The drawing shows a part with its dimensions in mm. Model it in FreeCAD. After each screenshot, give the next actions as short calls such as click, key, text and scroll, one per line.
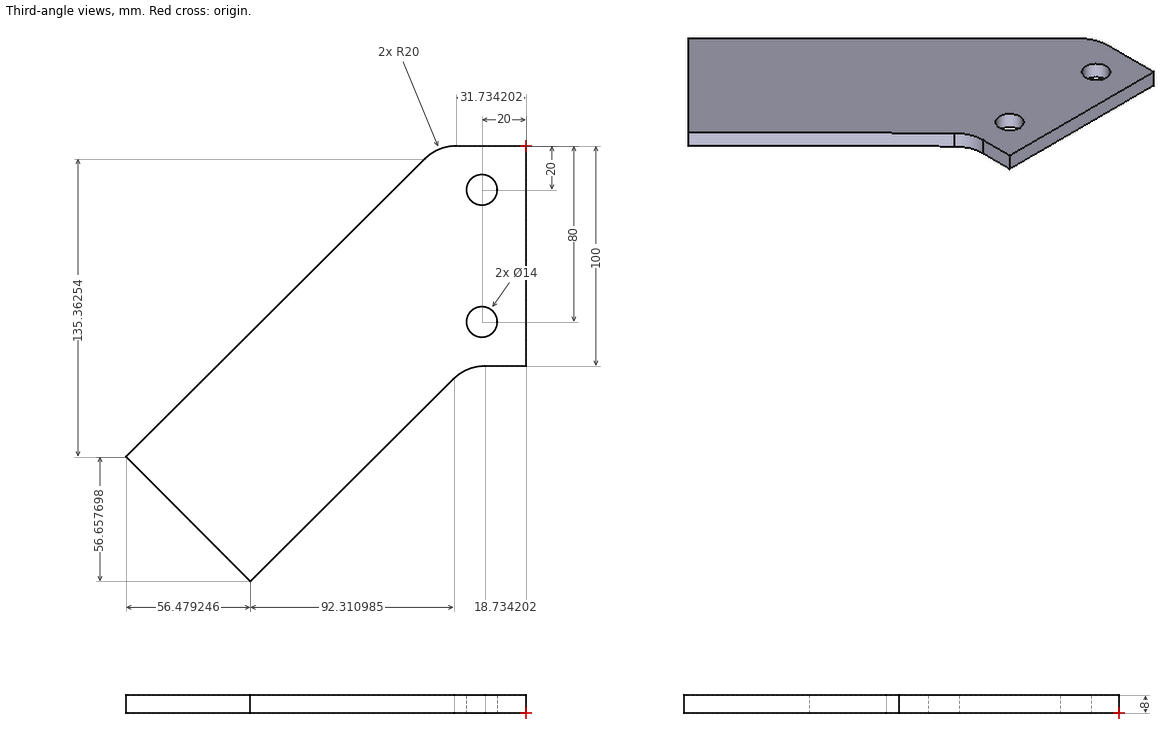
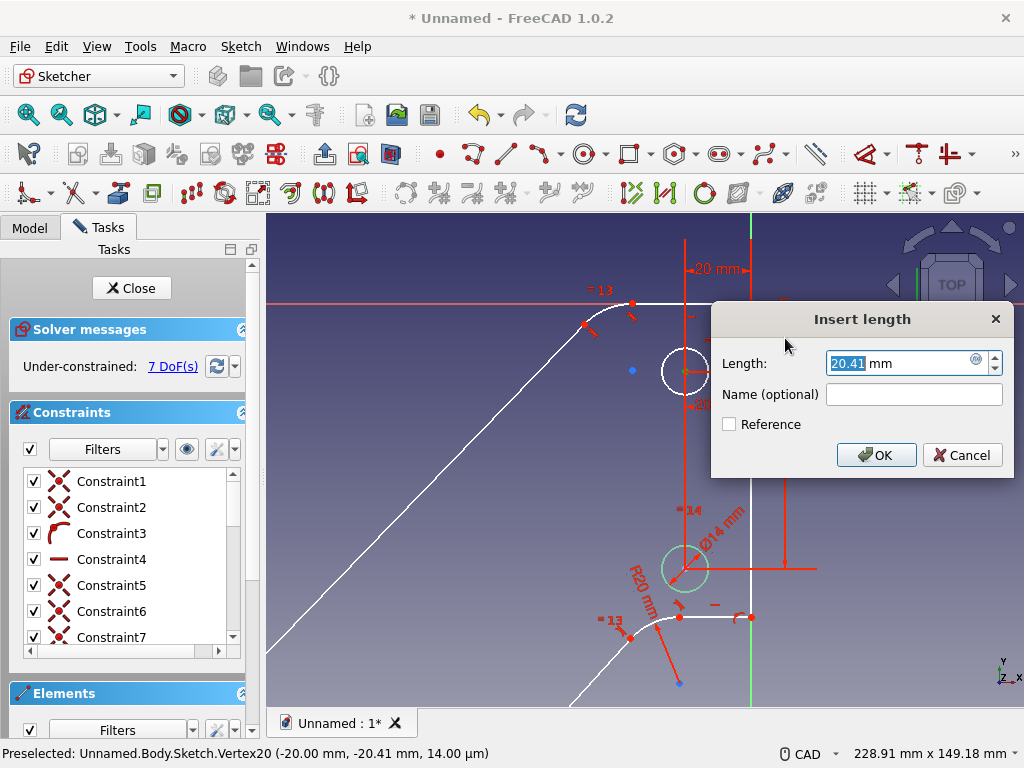
text(20)
key(Return)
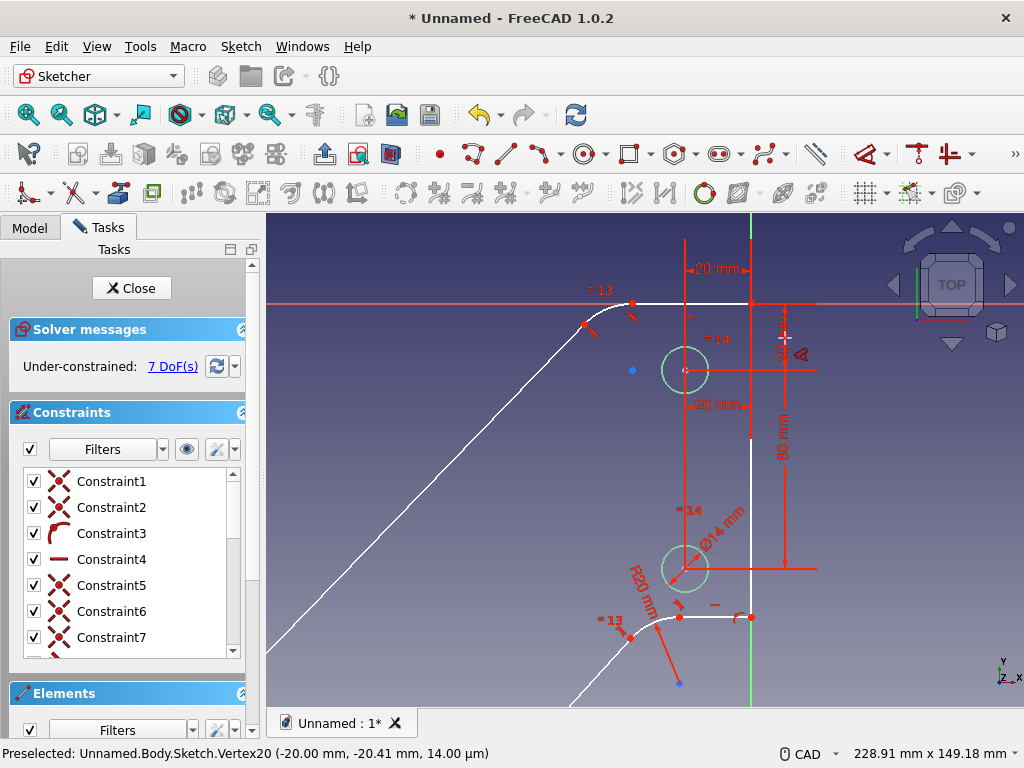
click(751, 523)
click(785, 461)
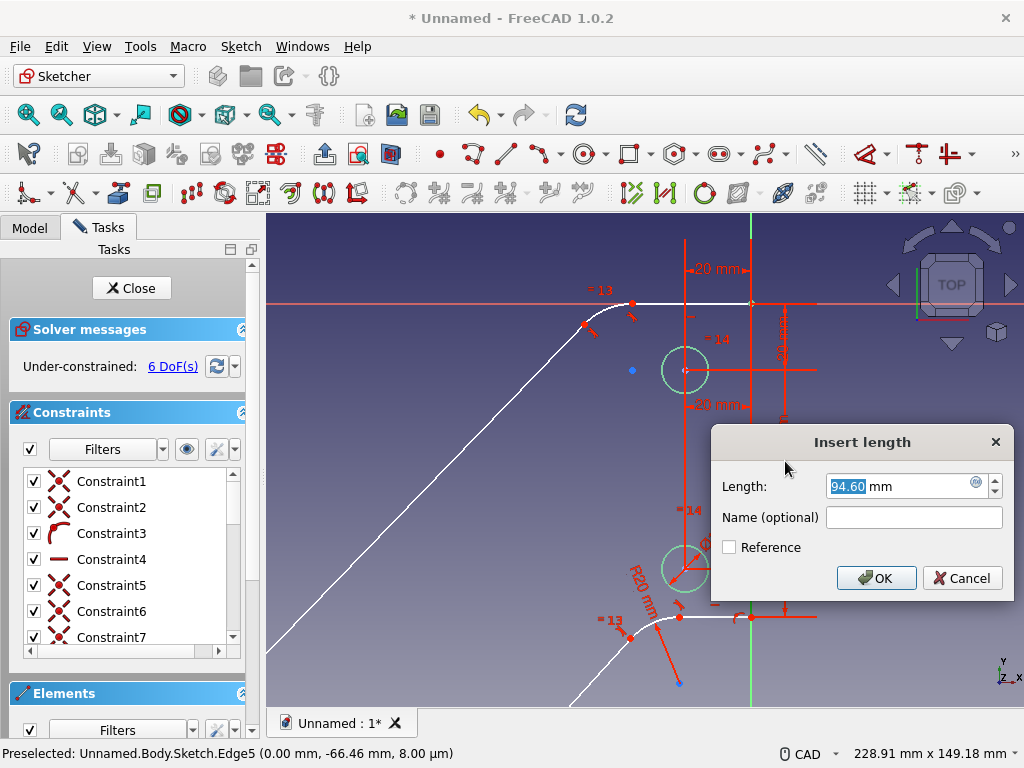
text(100)
key(Return)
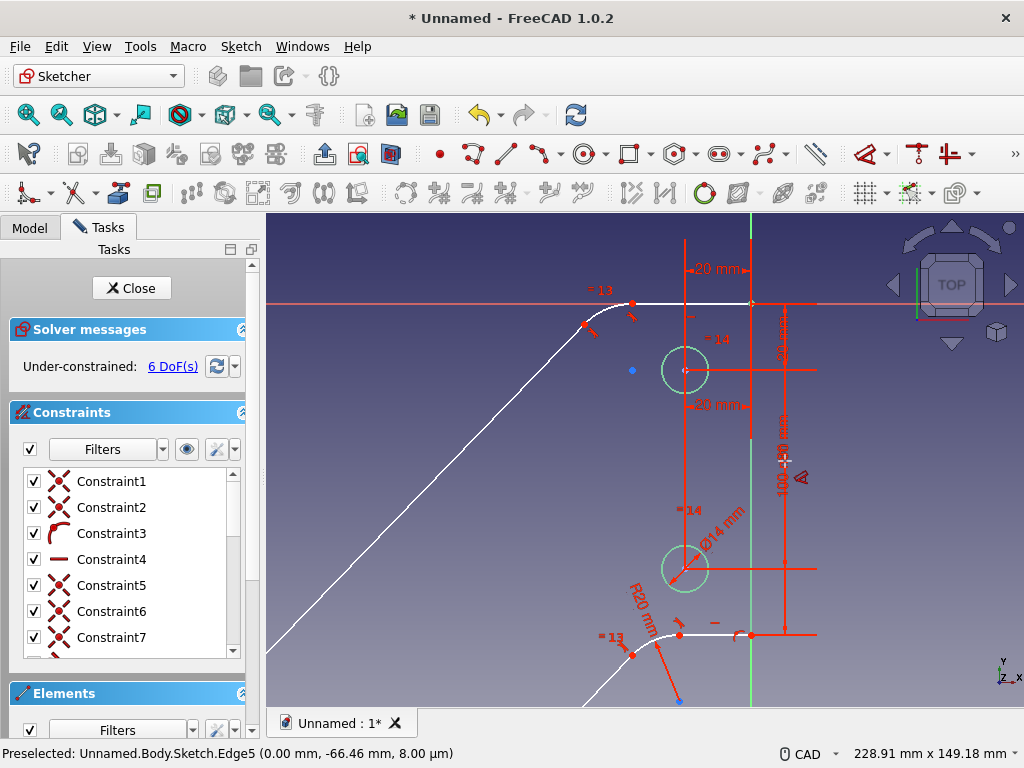
click(701, 635)
click(716, 669)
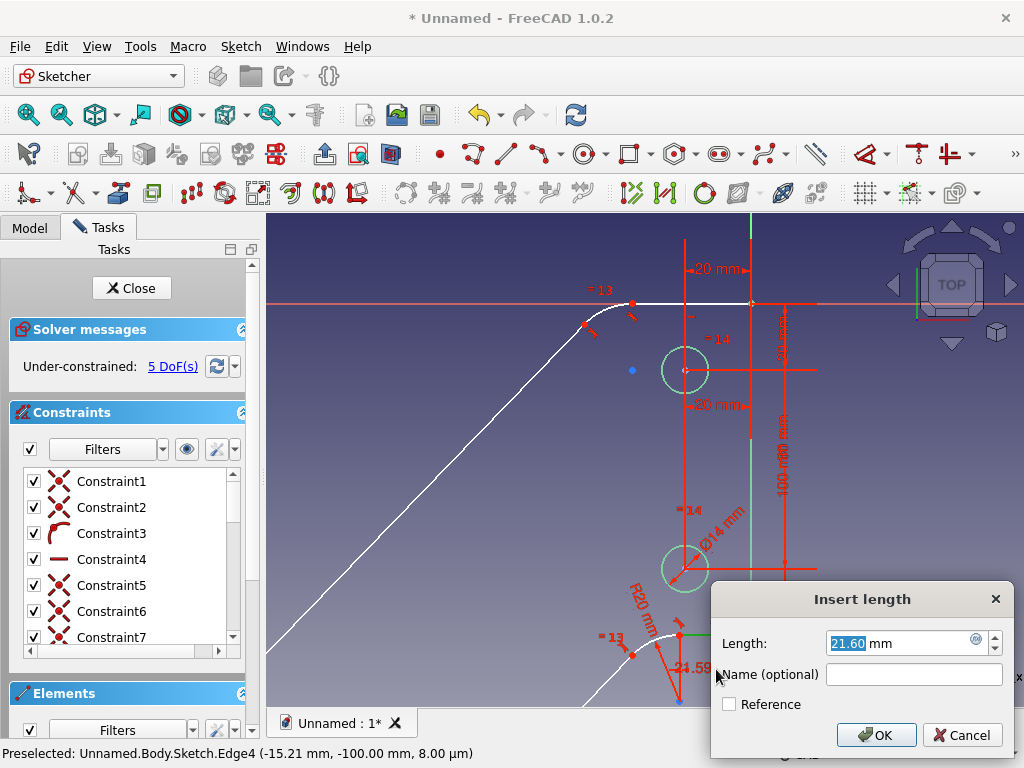
text(18.734202)
key(Return)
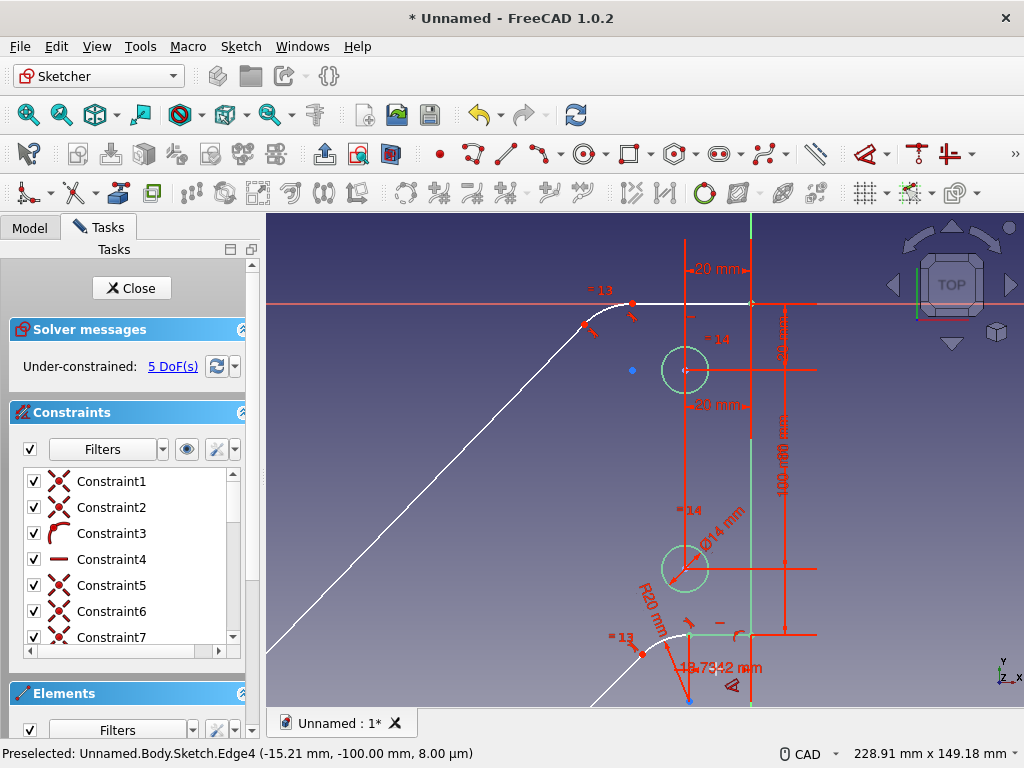
click(716, 304)
click(664, 338)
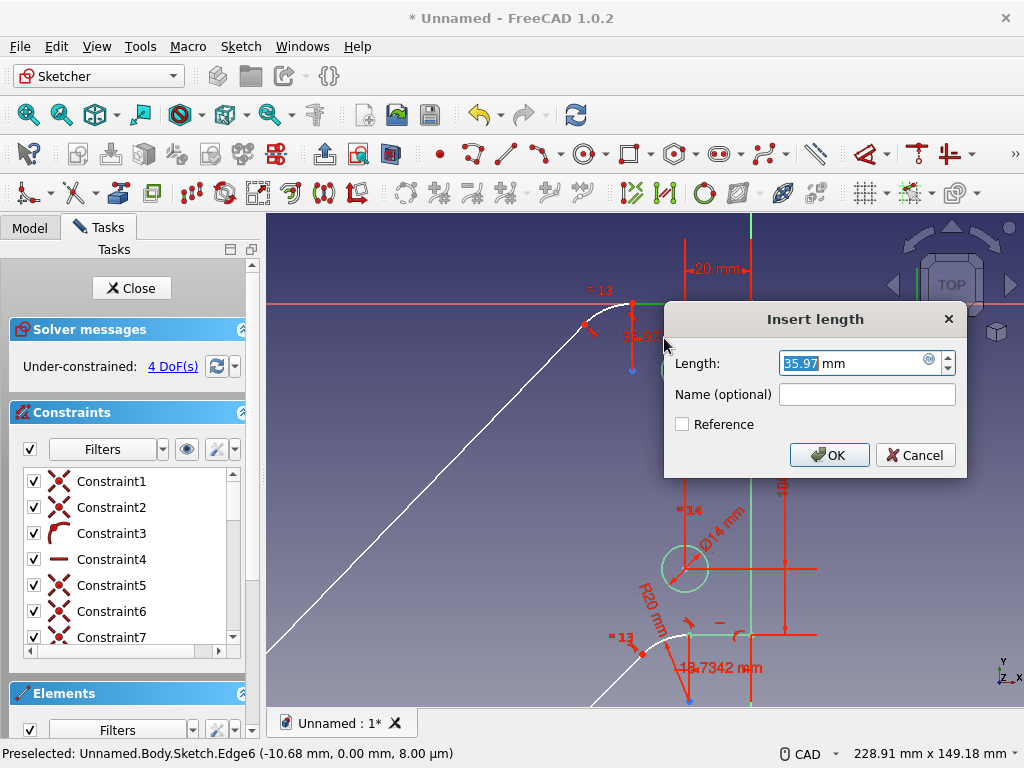
text(31.734202)
key(Return)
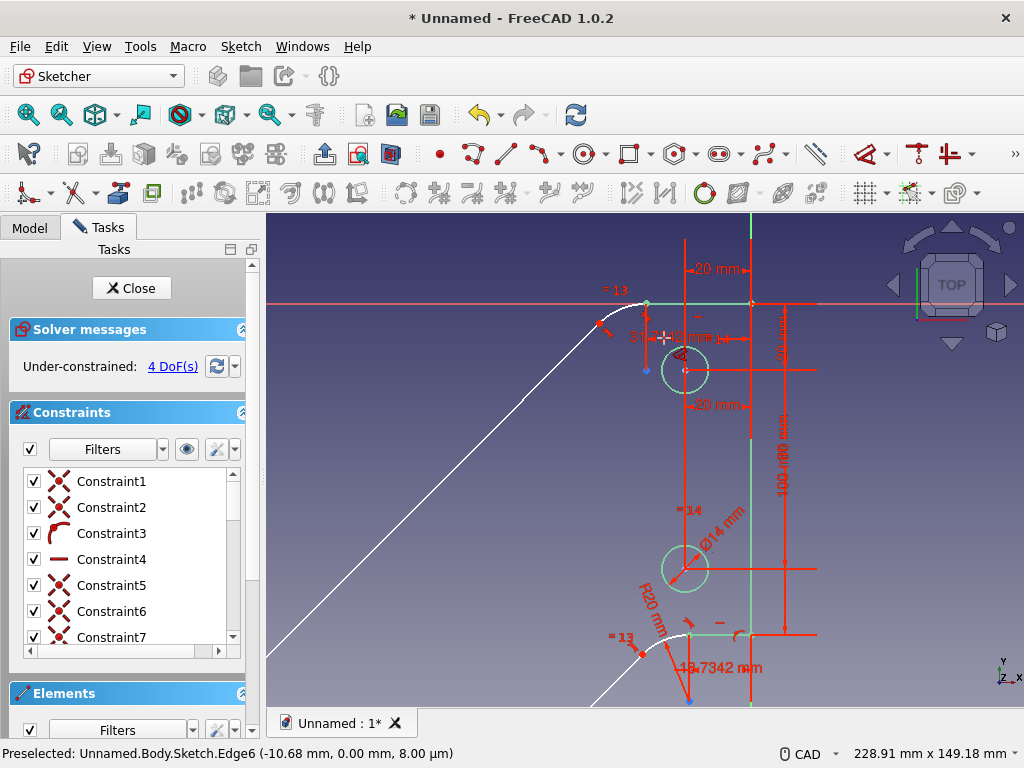
click(465, 458)
click(633, 501)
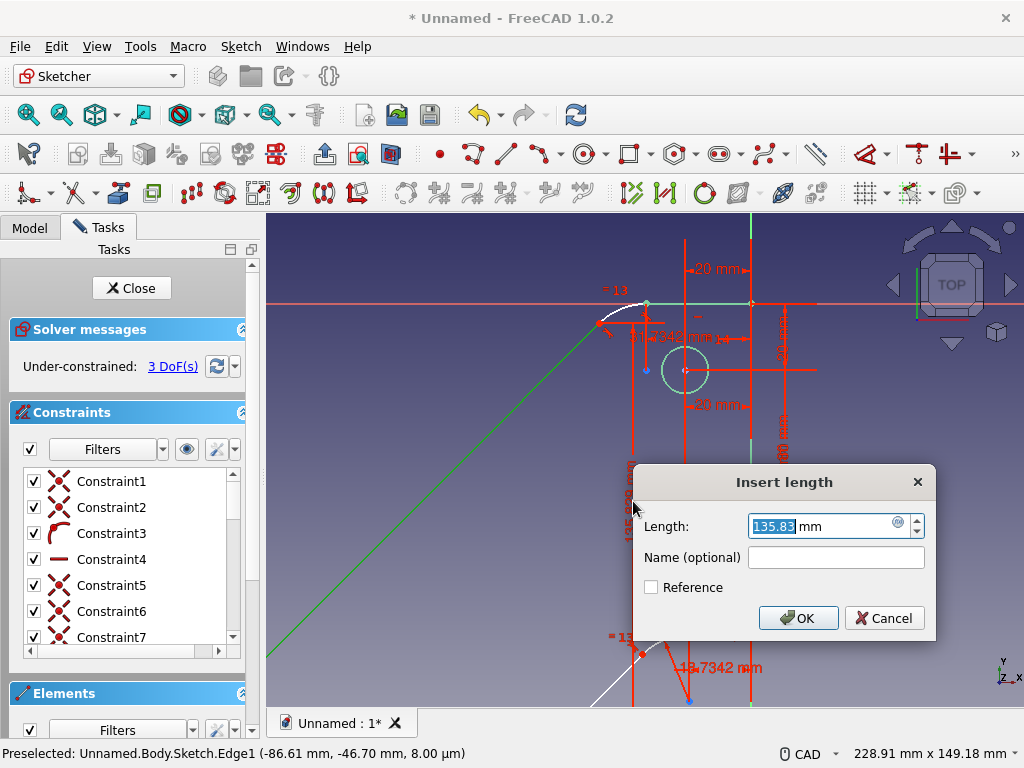
text(135.36254)
key(Return)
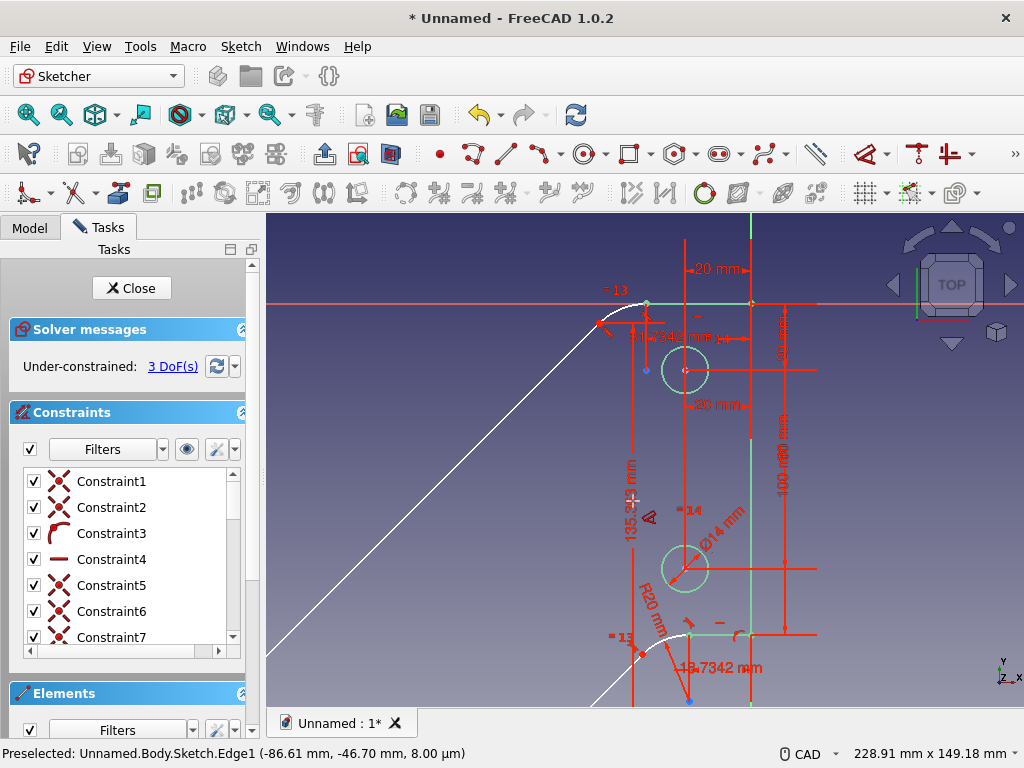
scroll(679, 320, down, 4)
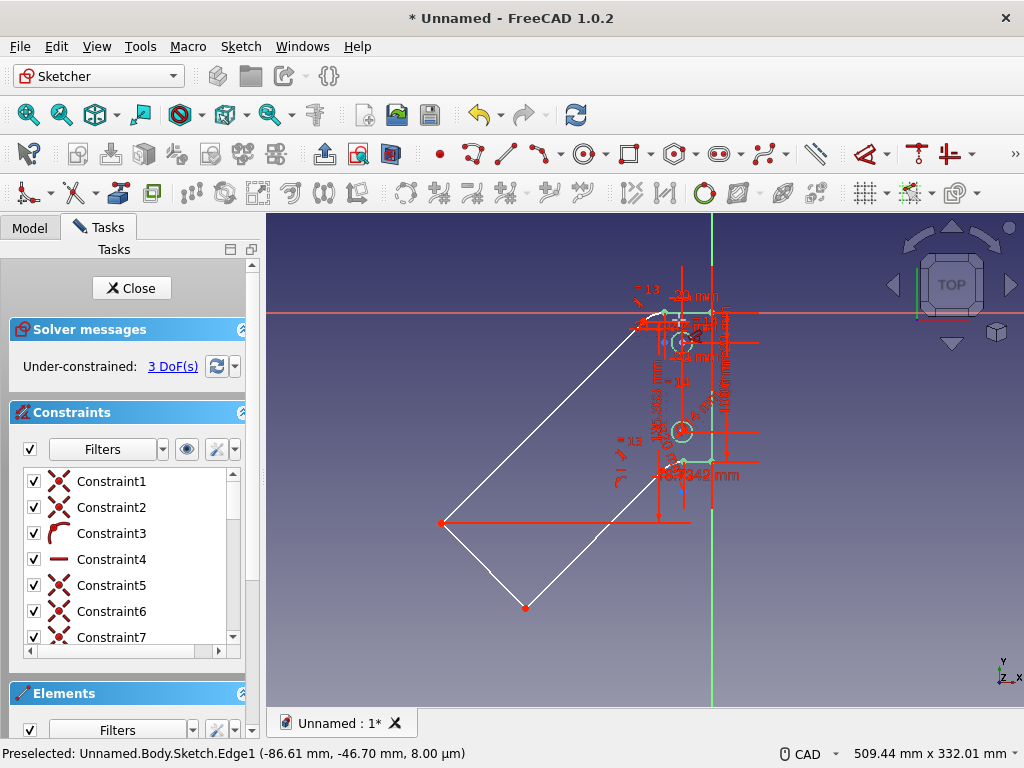
click(467, 549)
click(484, 643)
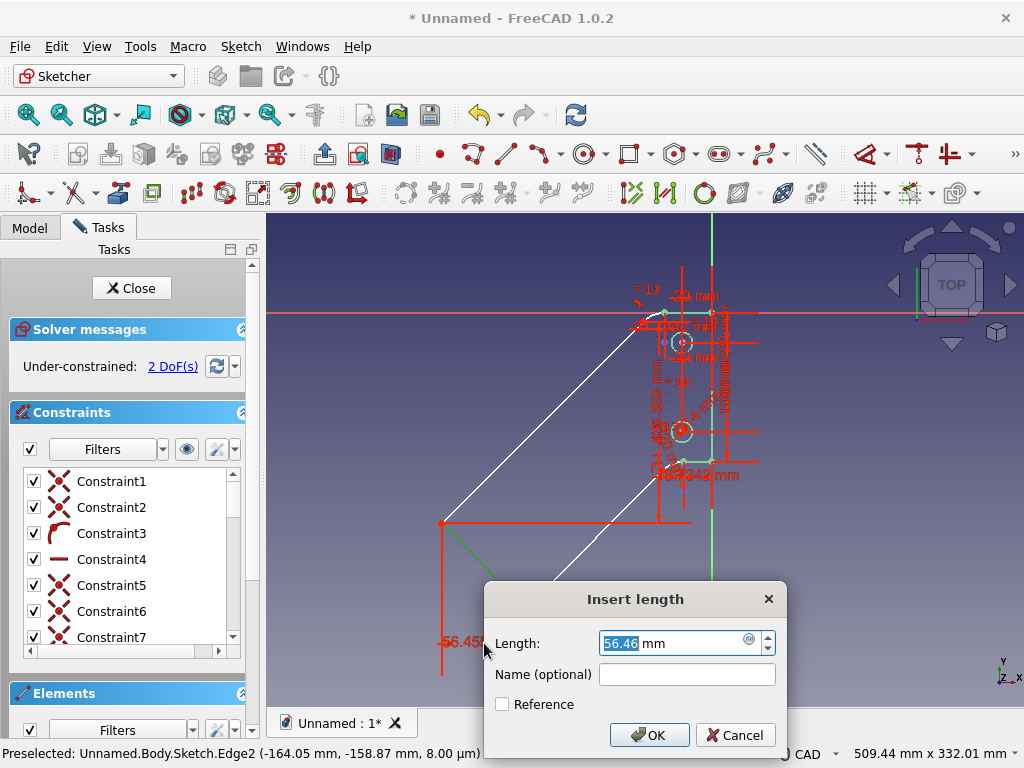
text(56.479246)
key(Return)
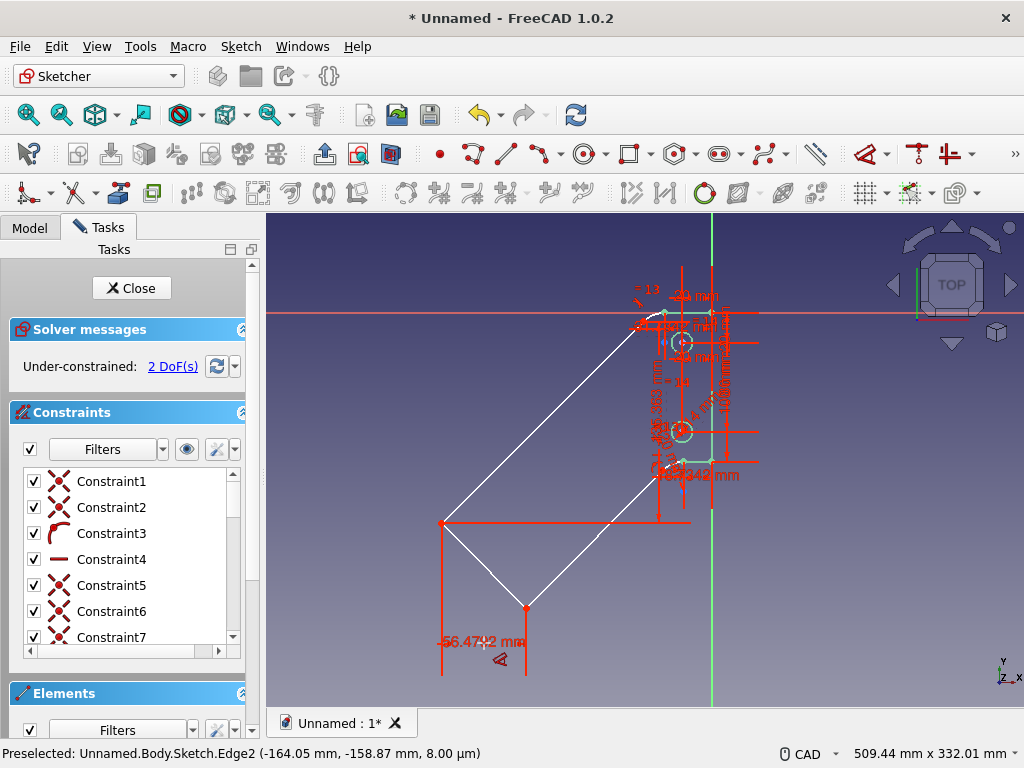
click(467, 549)
click(408, 566)